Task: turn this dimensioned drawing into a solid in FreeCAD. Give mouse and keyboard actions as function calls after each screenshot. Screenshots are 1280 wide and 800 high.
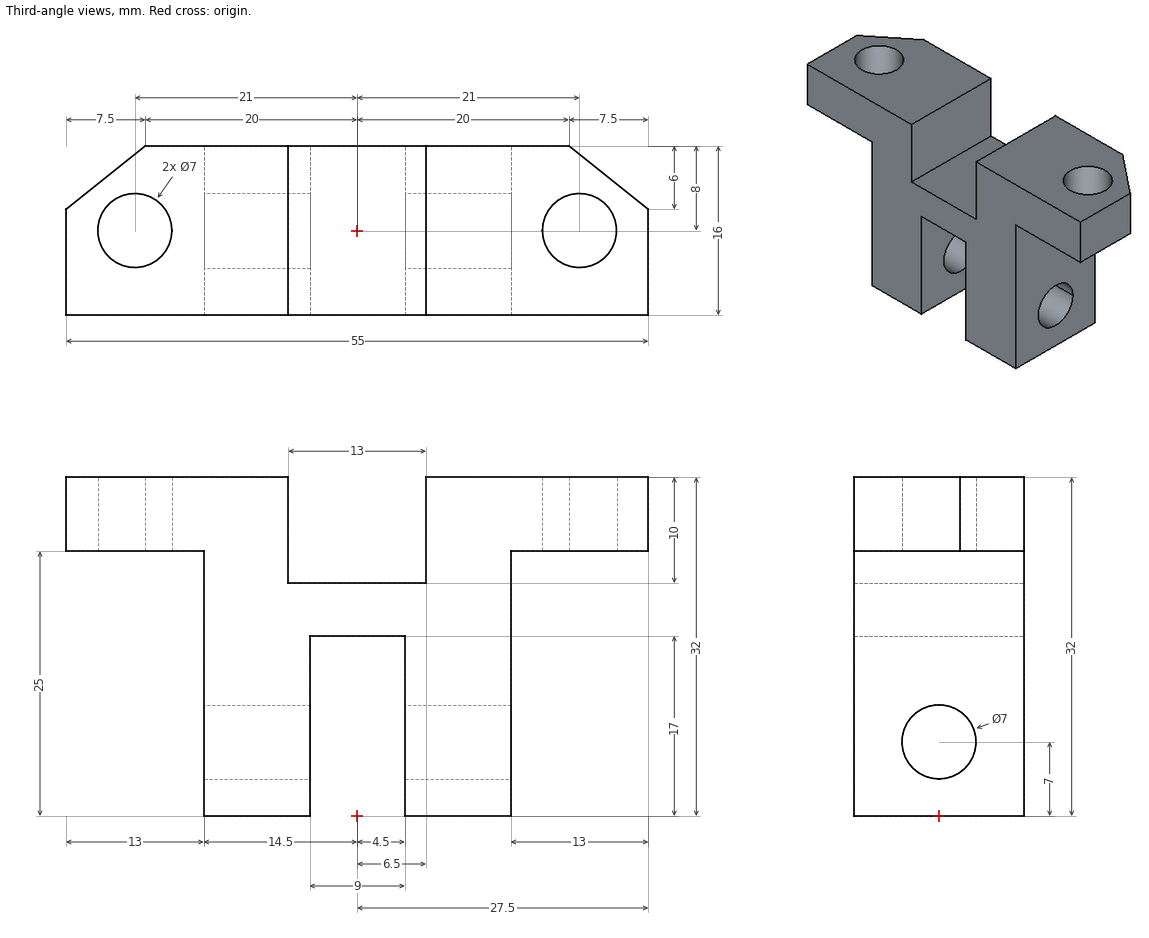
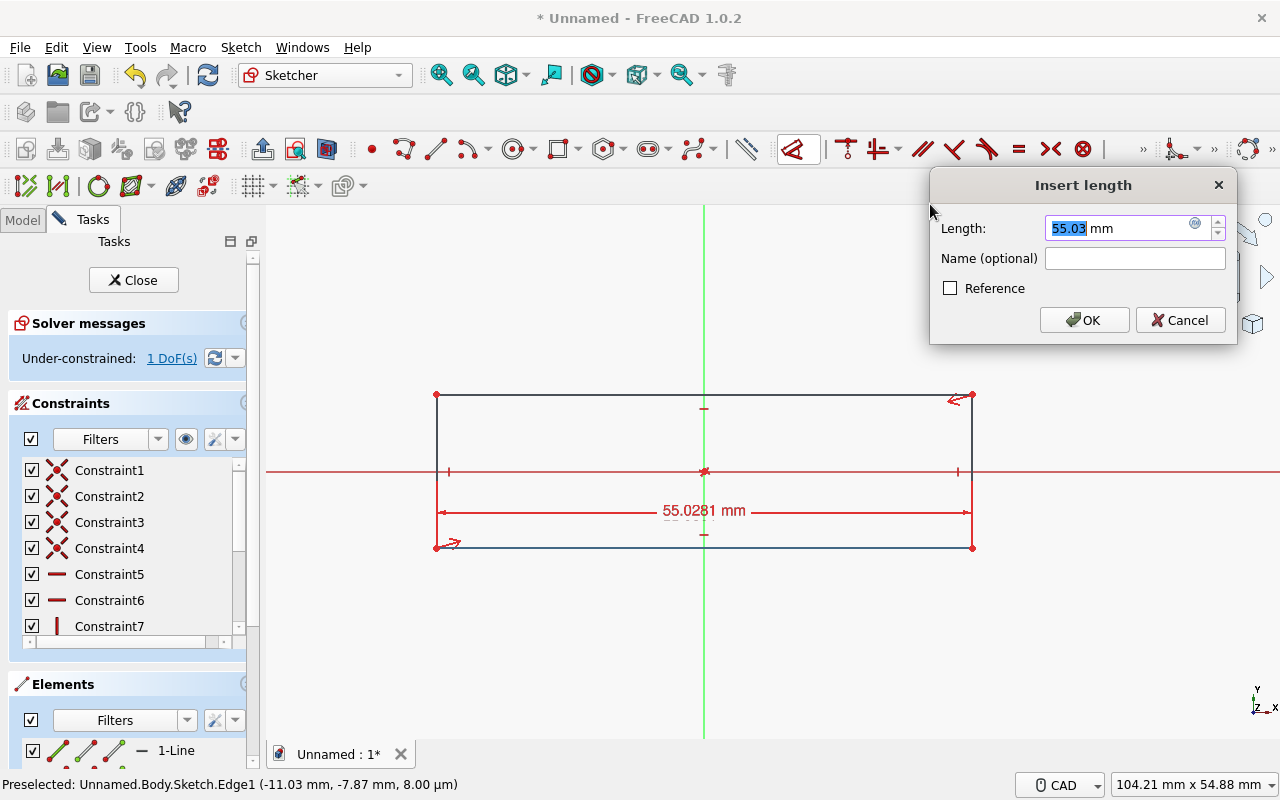
text(55)
key(Return)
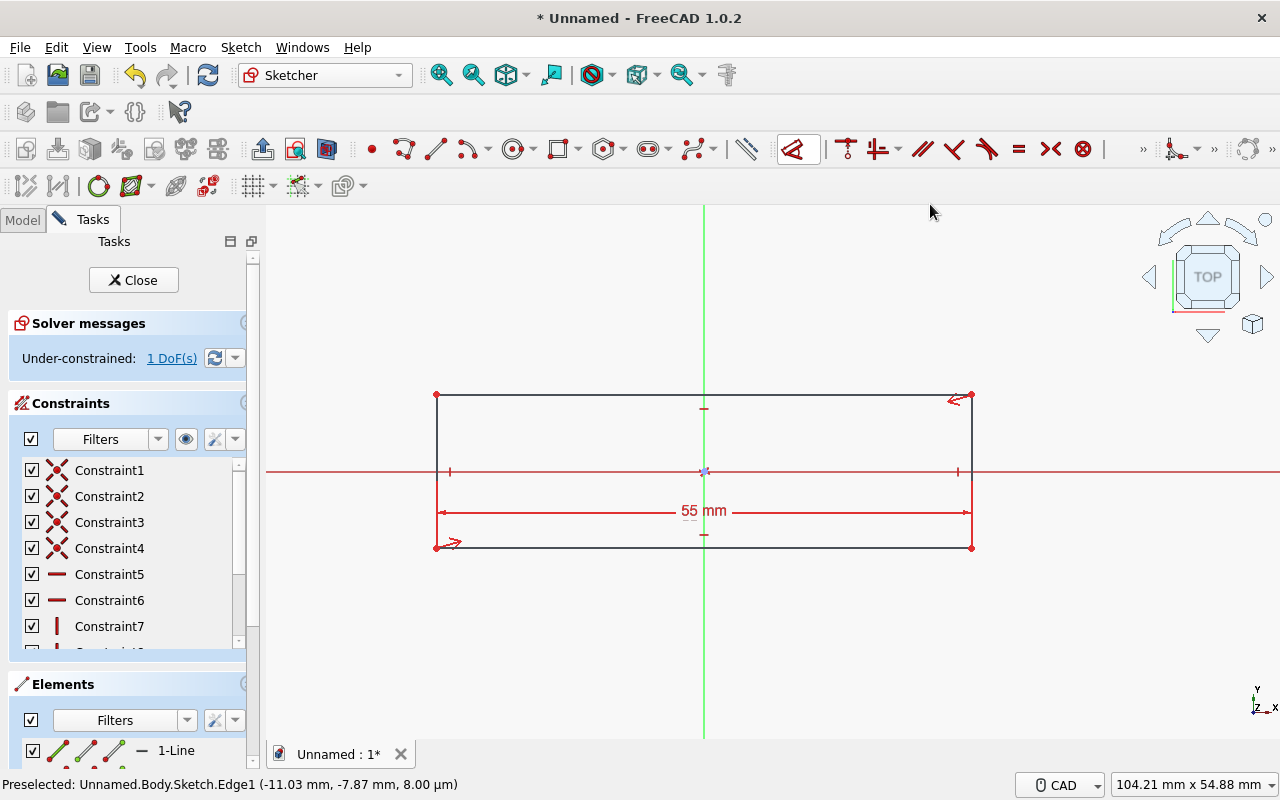
click(972, 502)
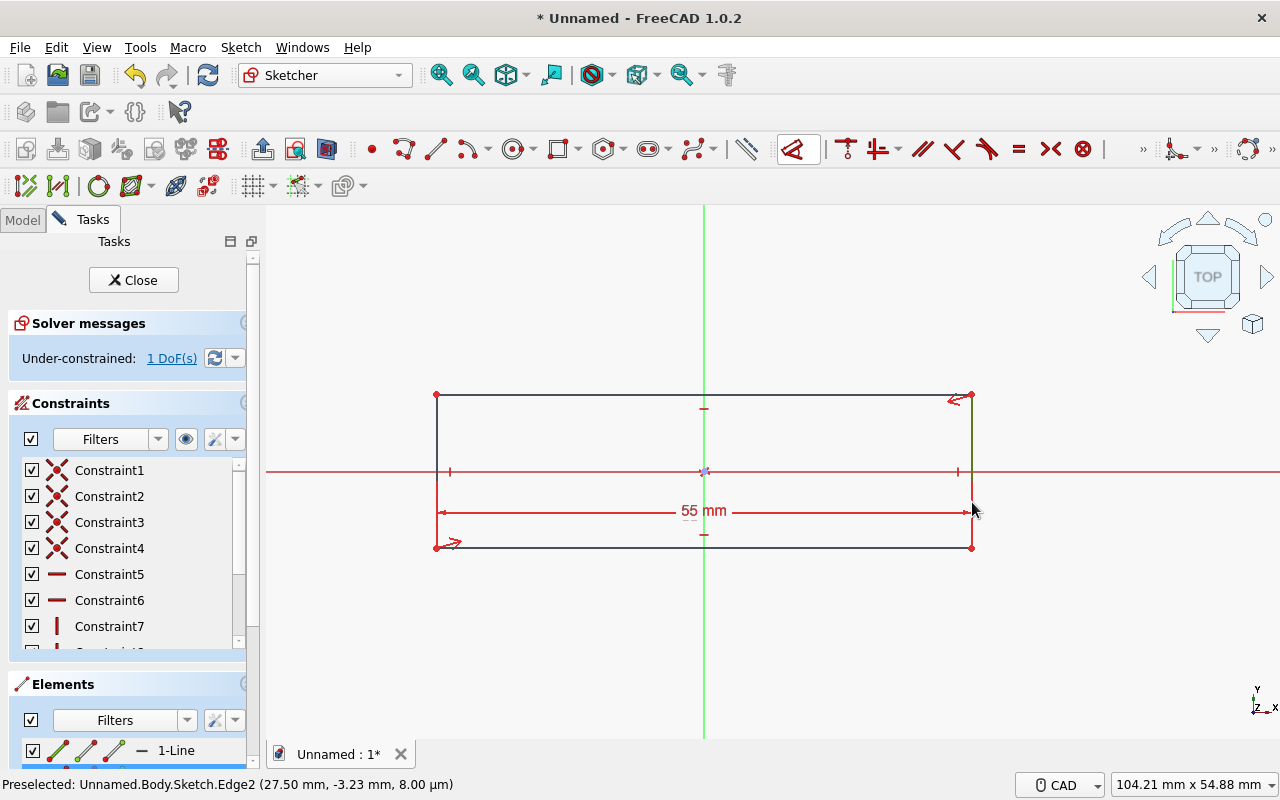
key(i)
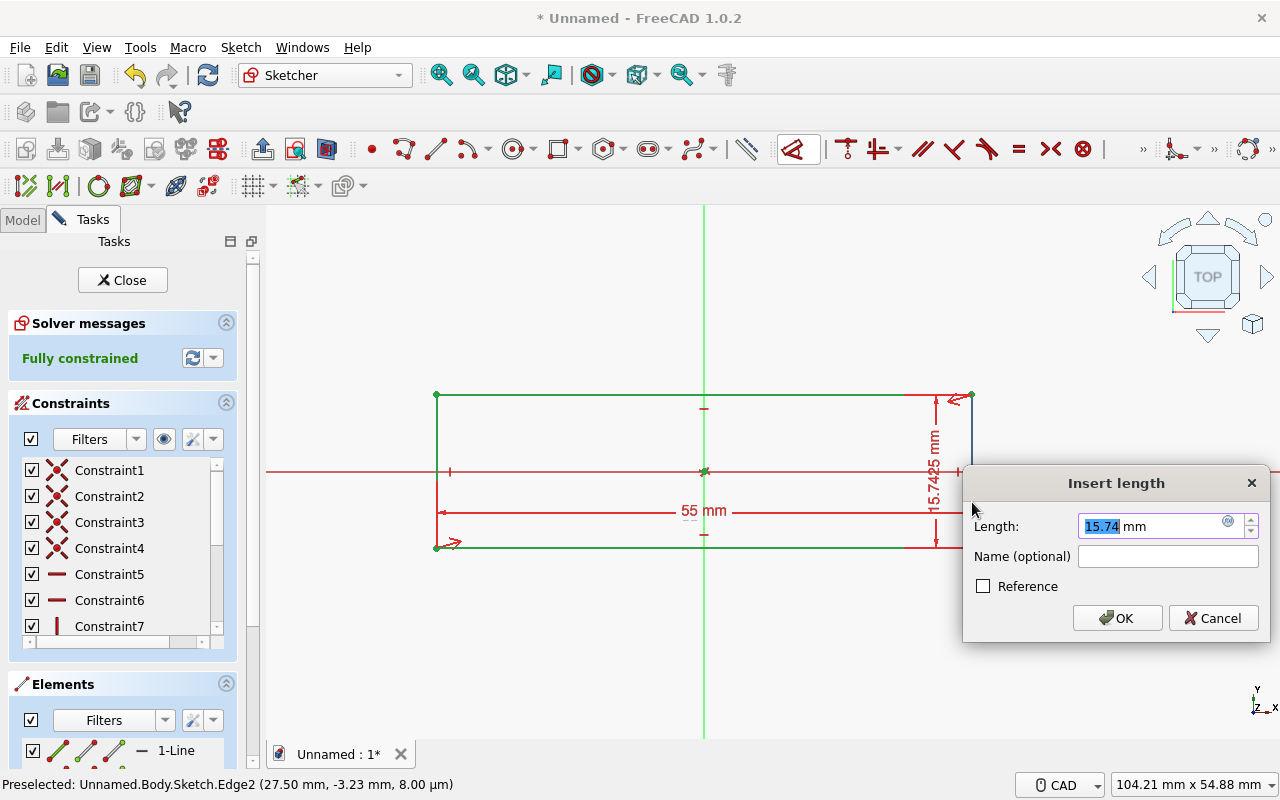
text(16)
key(Return)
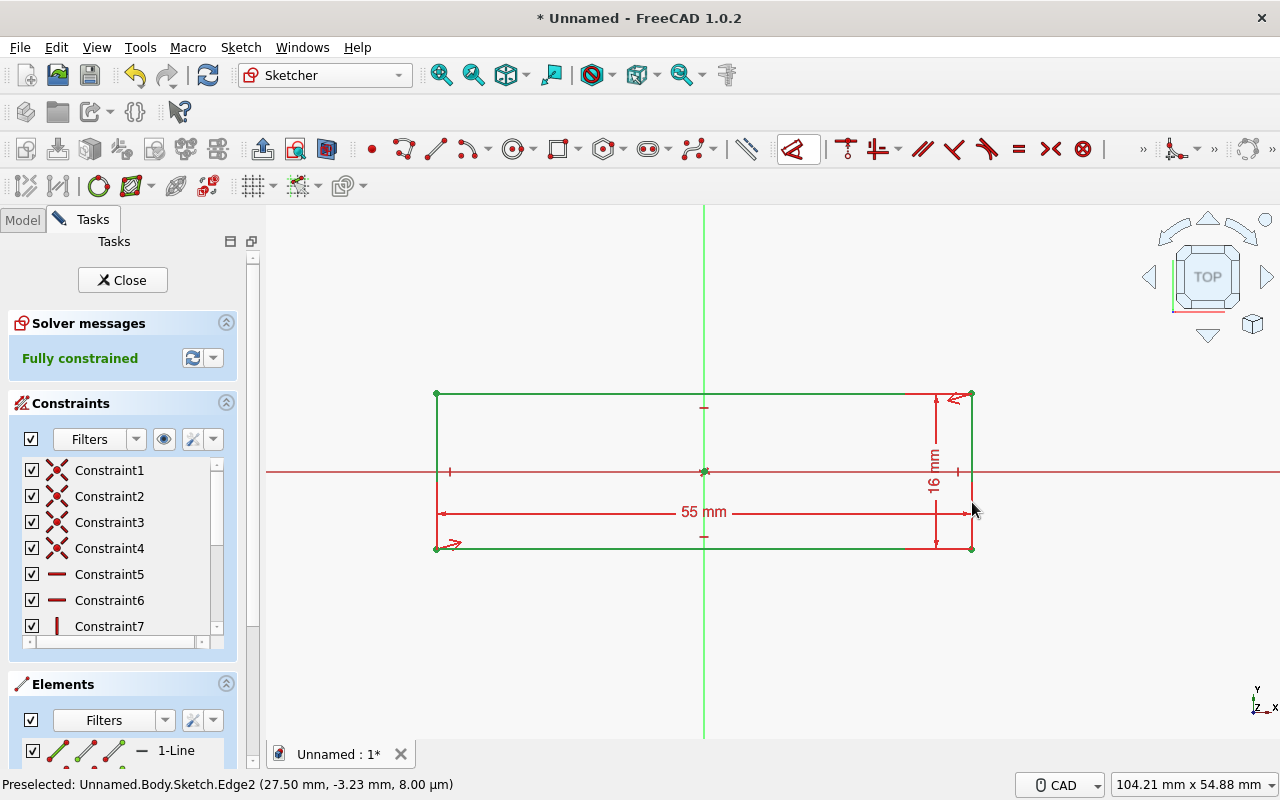
click(123, 280)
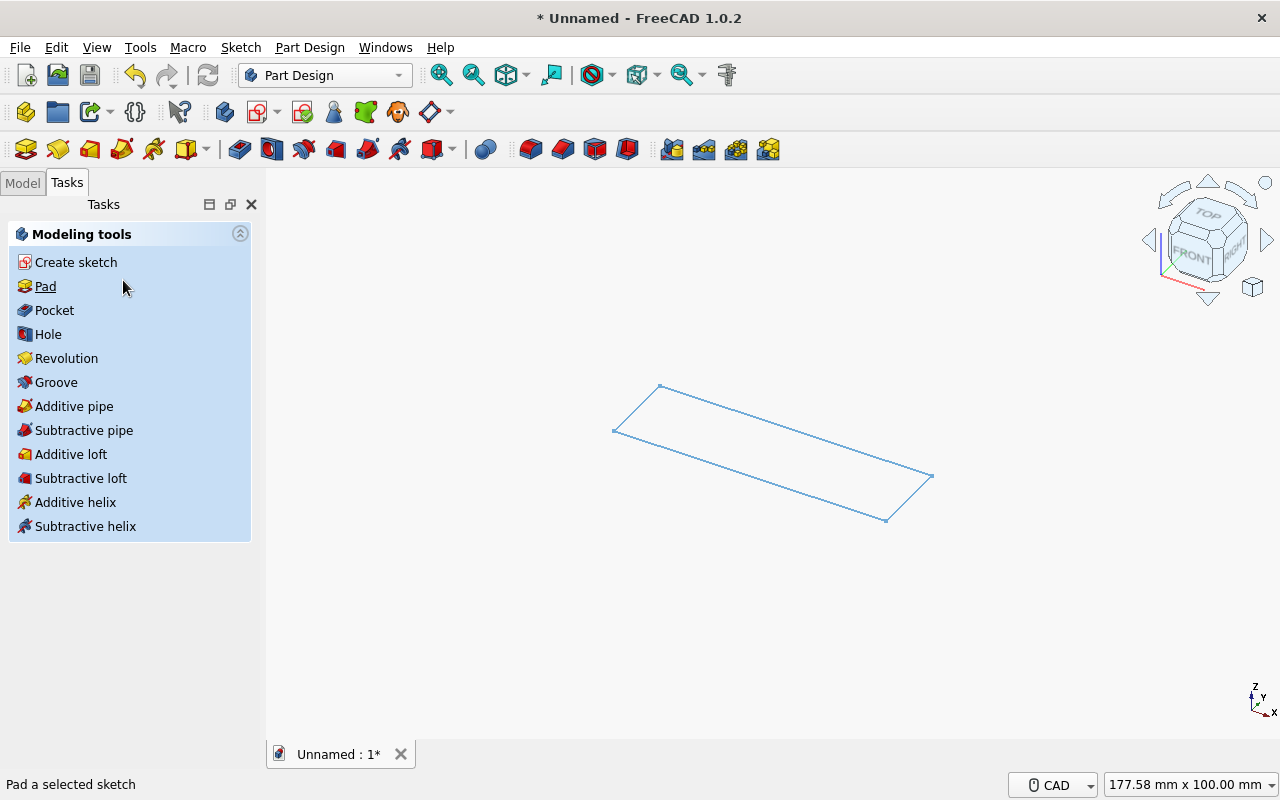
click(26, 150)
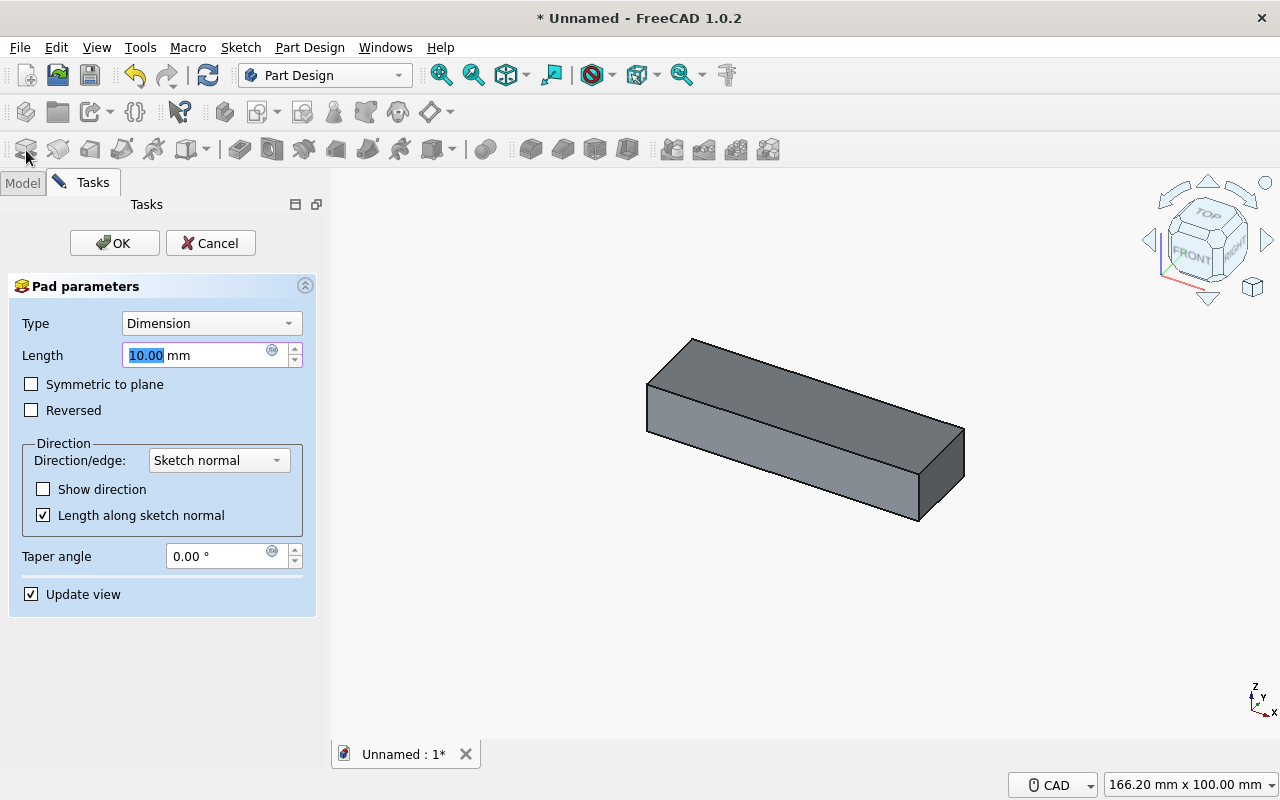
text(32)
key(Tab)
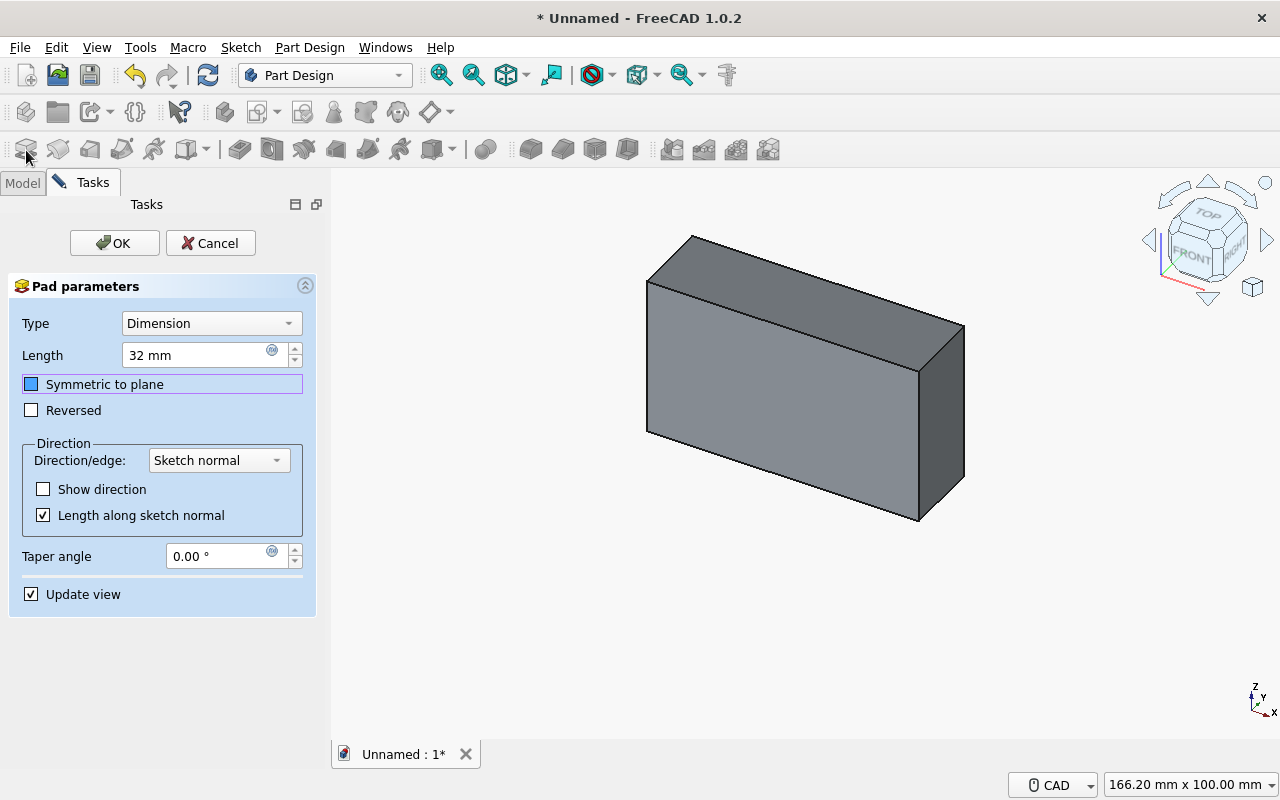
click(115, 243)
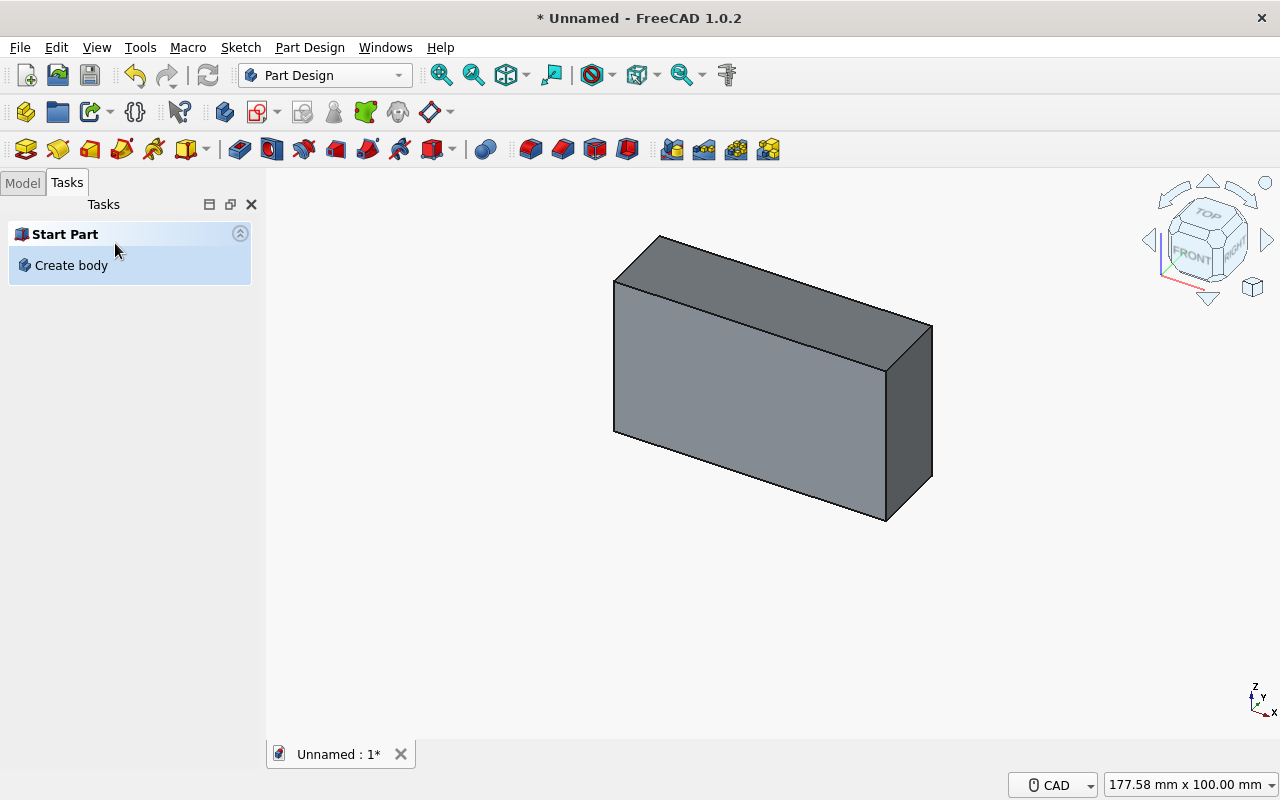
key(4)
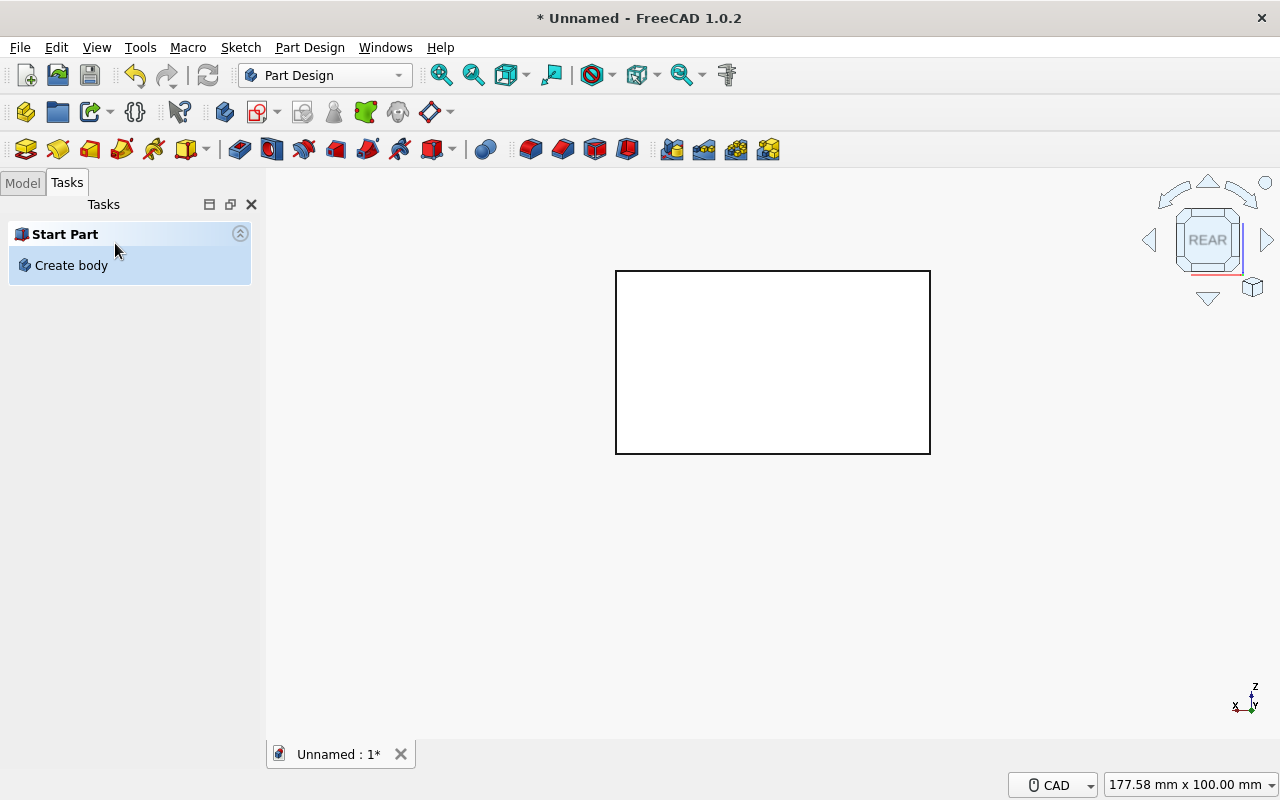
click(442, 76)